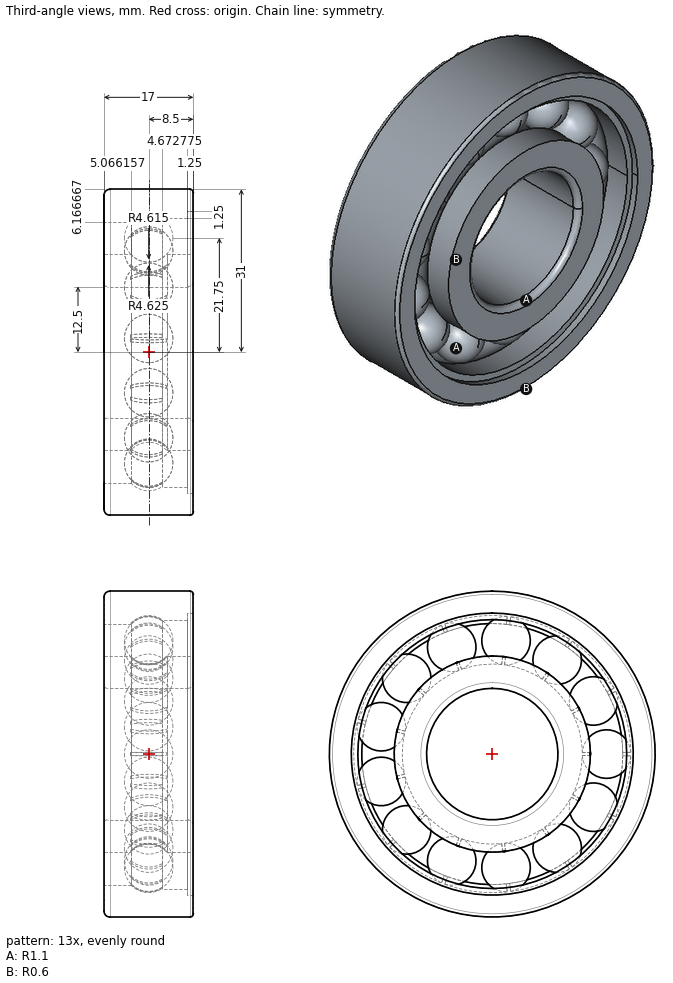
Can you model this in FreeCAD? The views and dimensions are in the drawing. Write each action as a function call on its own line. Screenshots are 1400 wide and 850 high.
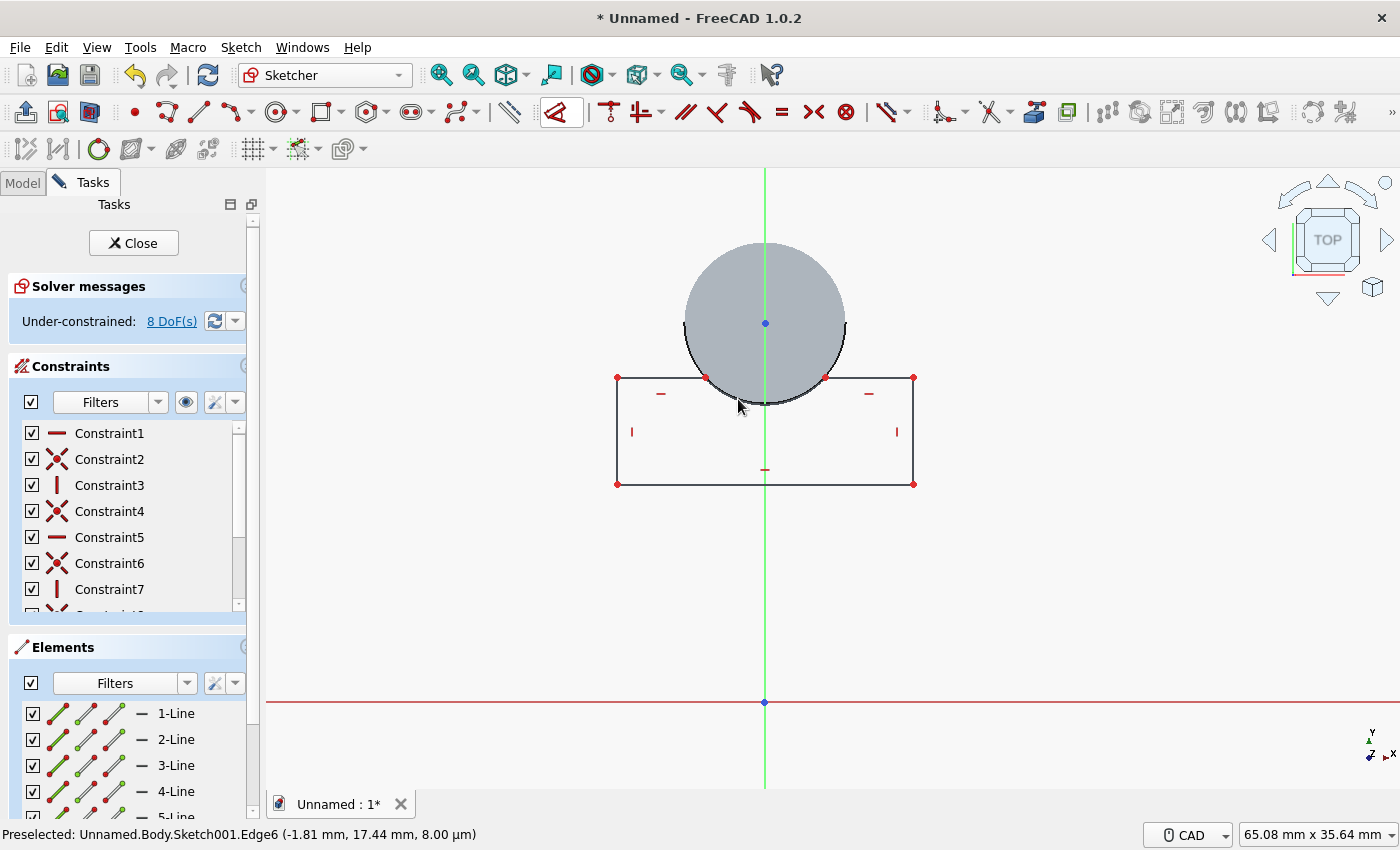
click(765, 324)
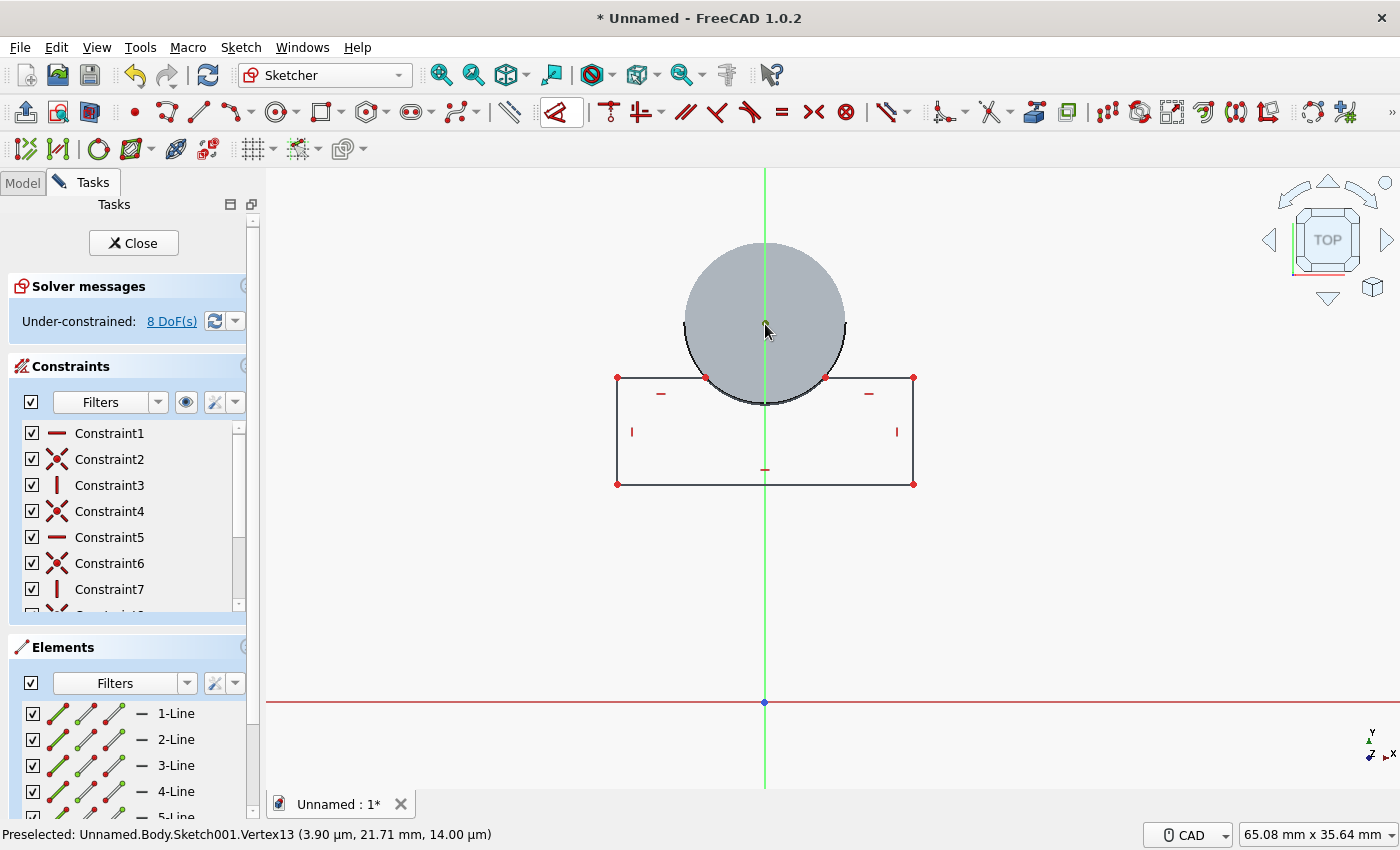
click(765, 640)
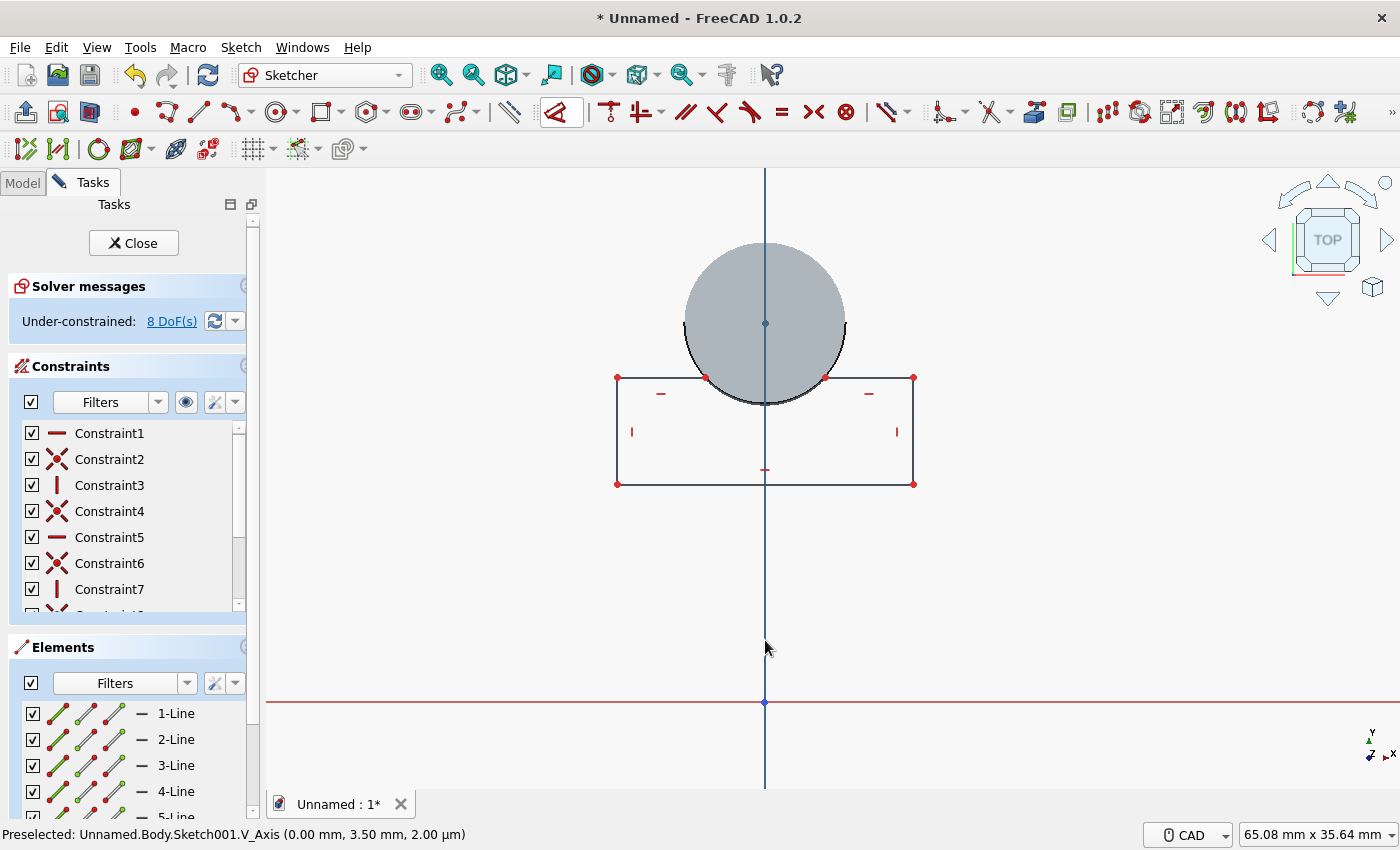
key(c)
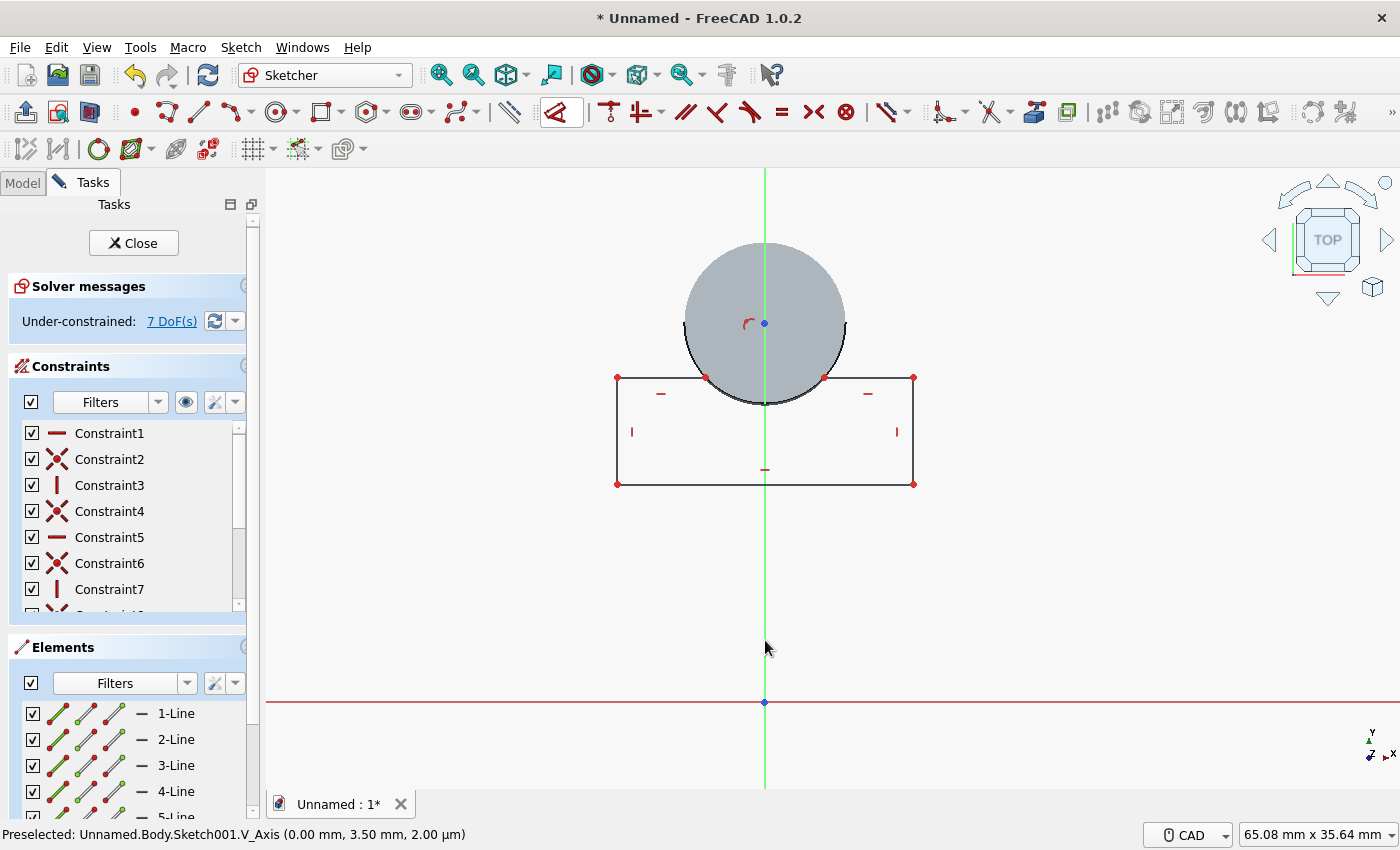
click(617, 378)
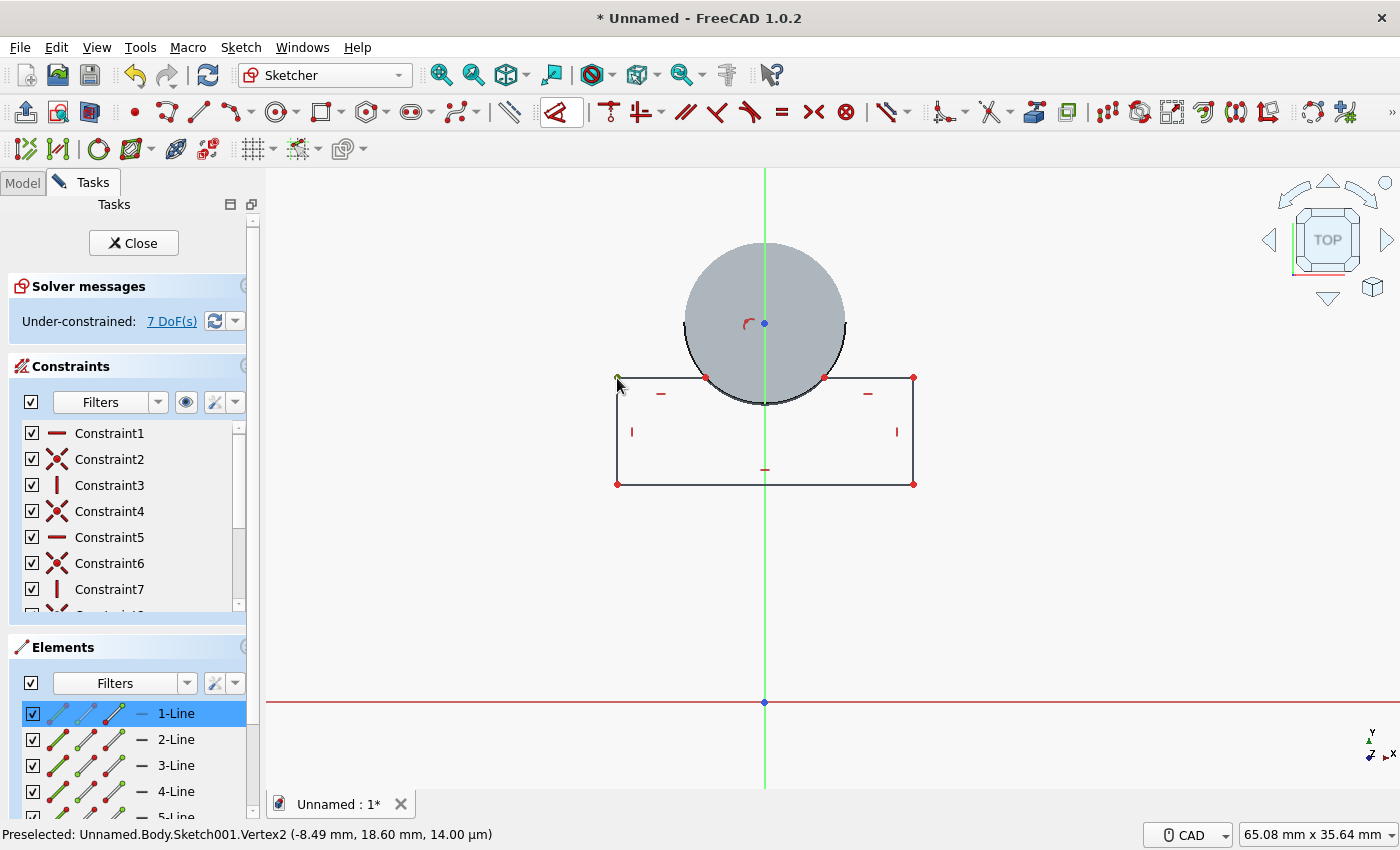
click(913, 378)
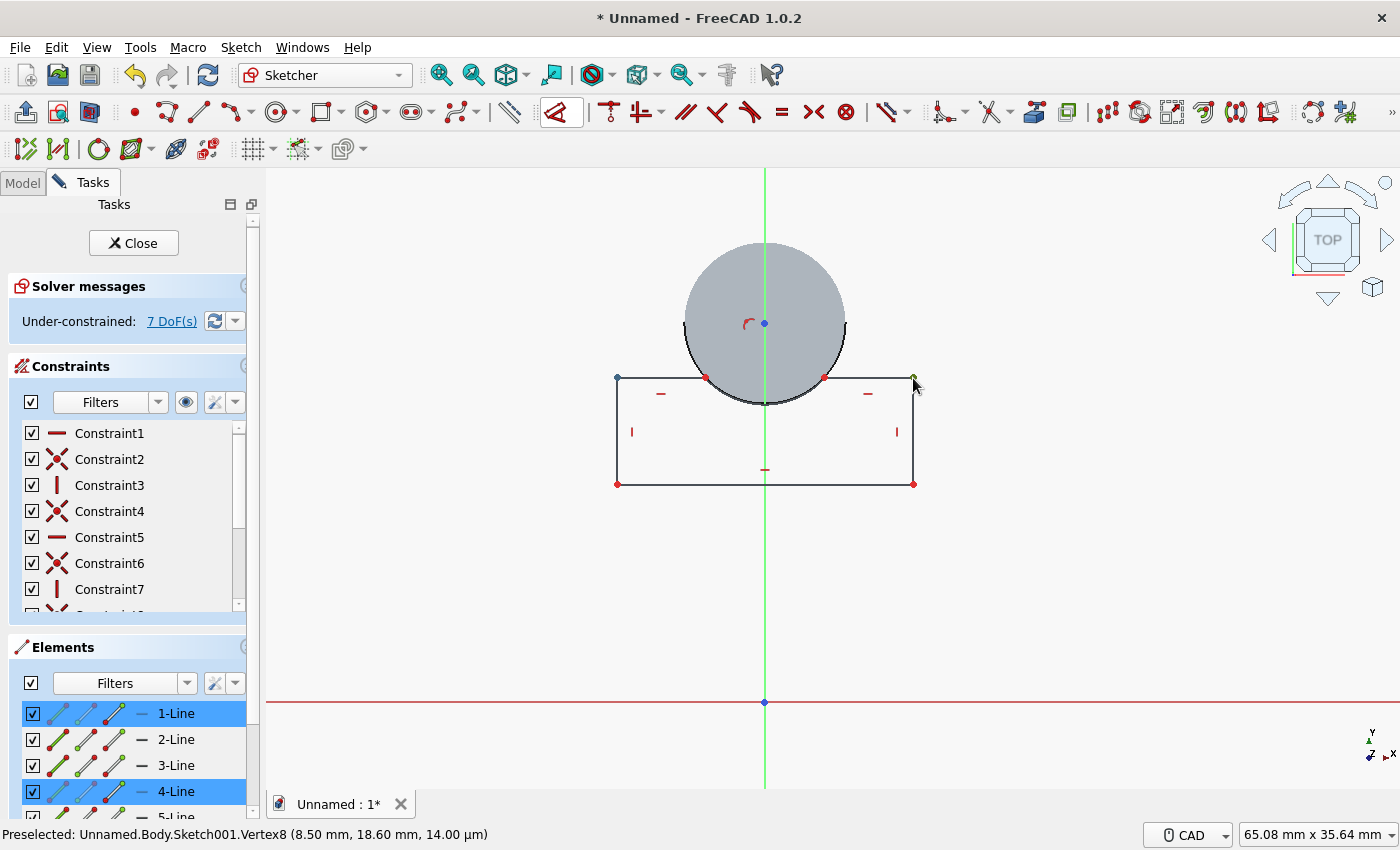
click(765, 640)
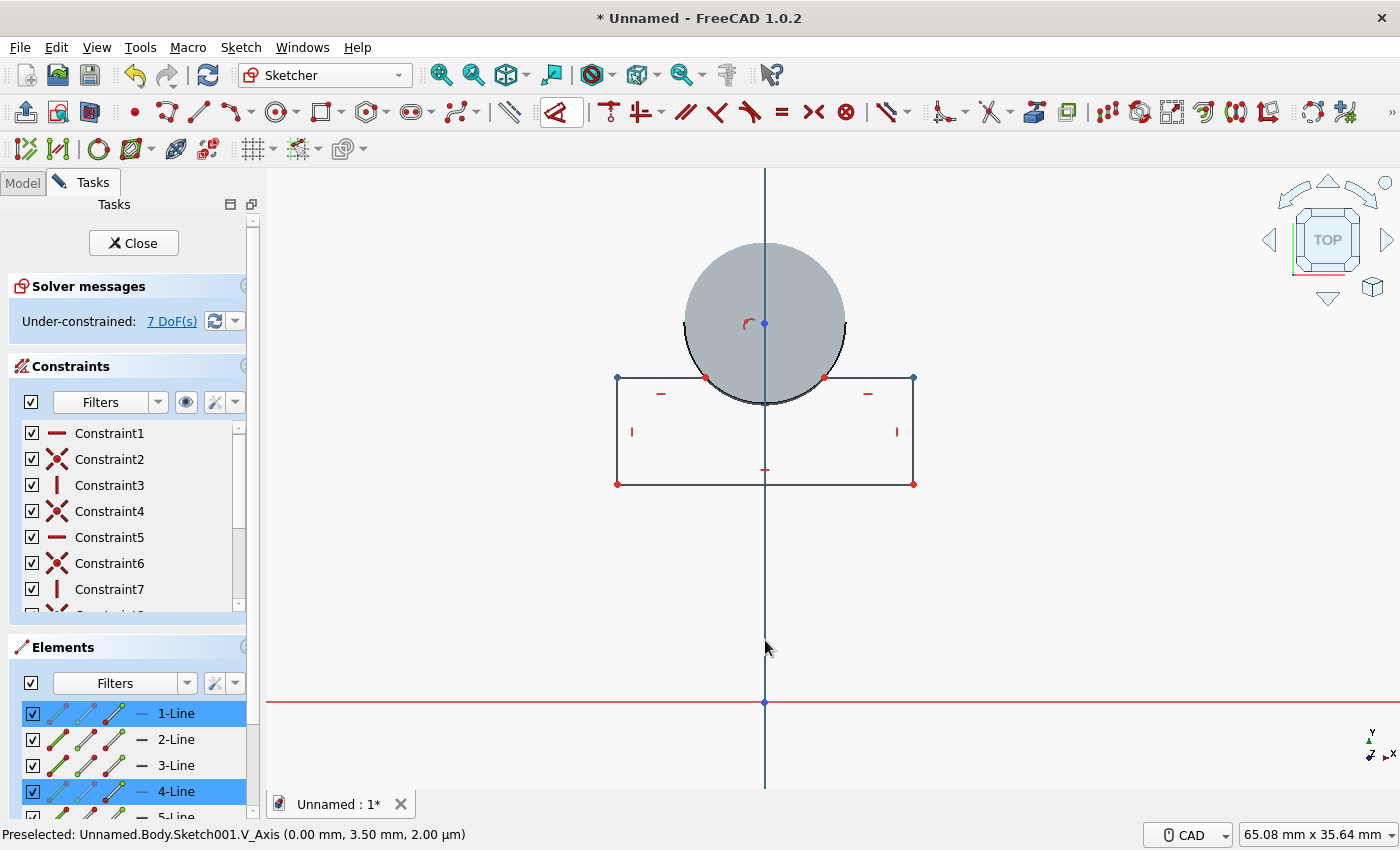
click(814, 112)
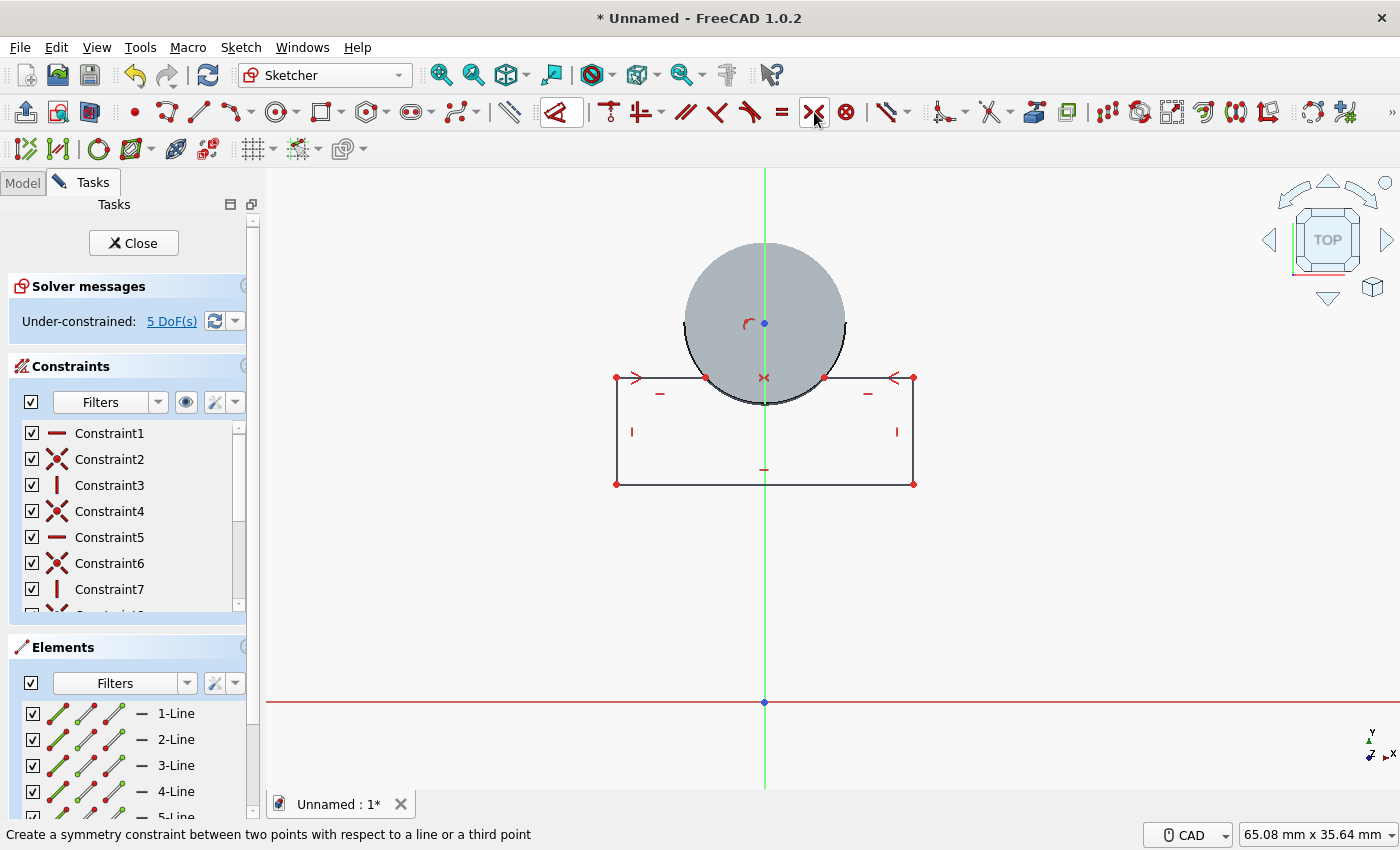
click(738, 400)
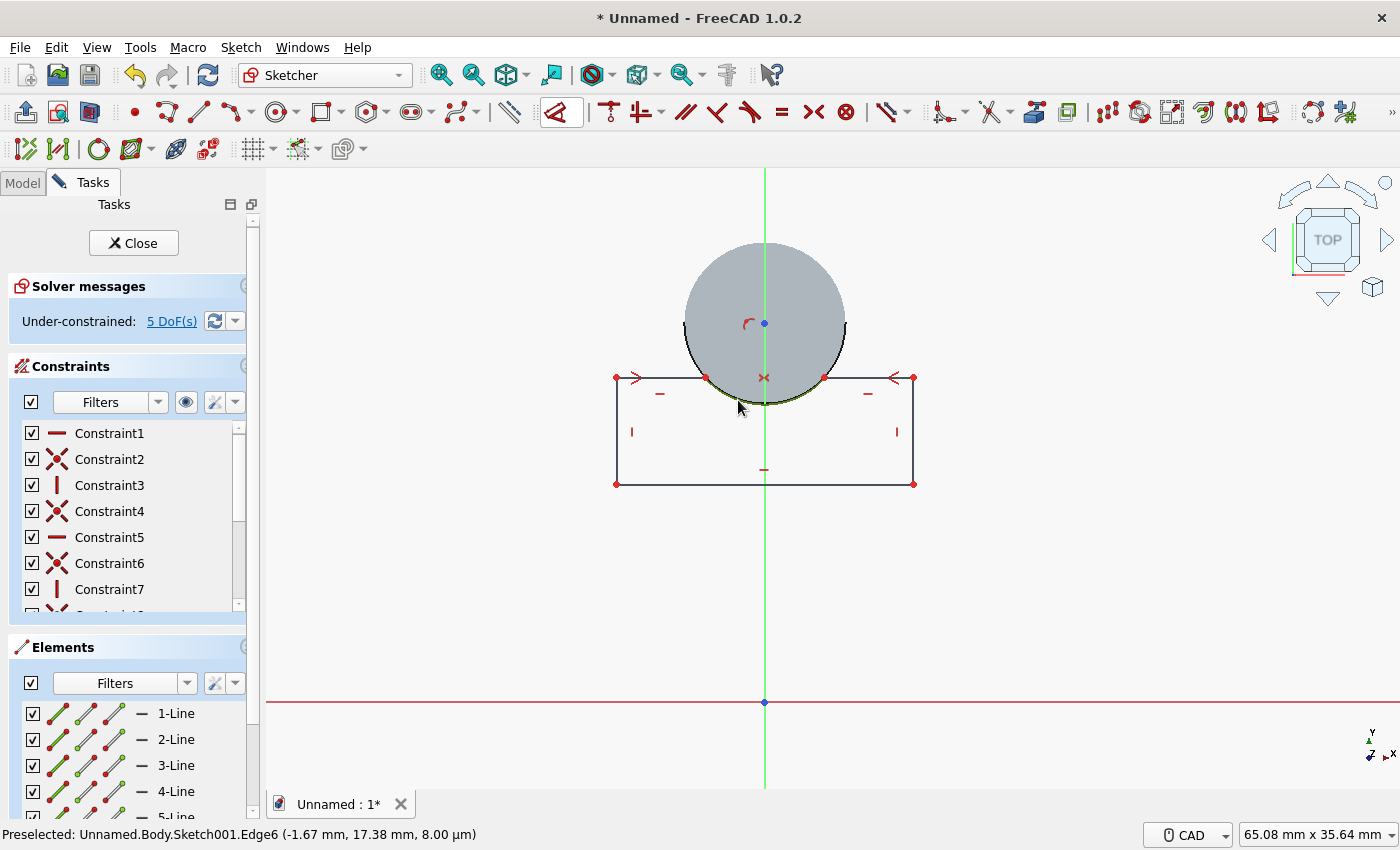
key(k)
key(r)